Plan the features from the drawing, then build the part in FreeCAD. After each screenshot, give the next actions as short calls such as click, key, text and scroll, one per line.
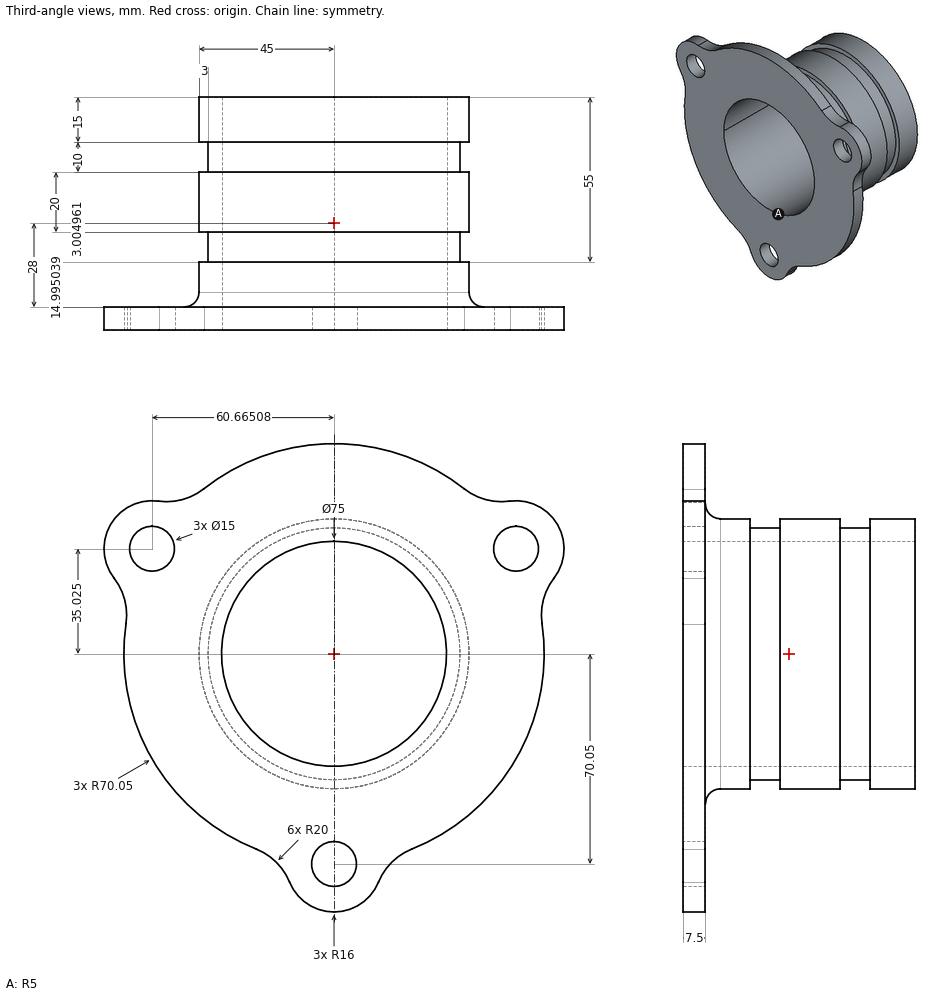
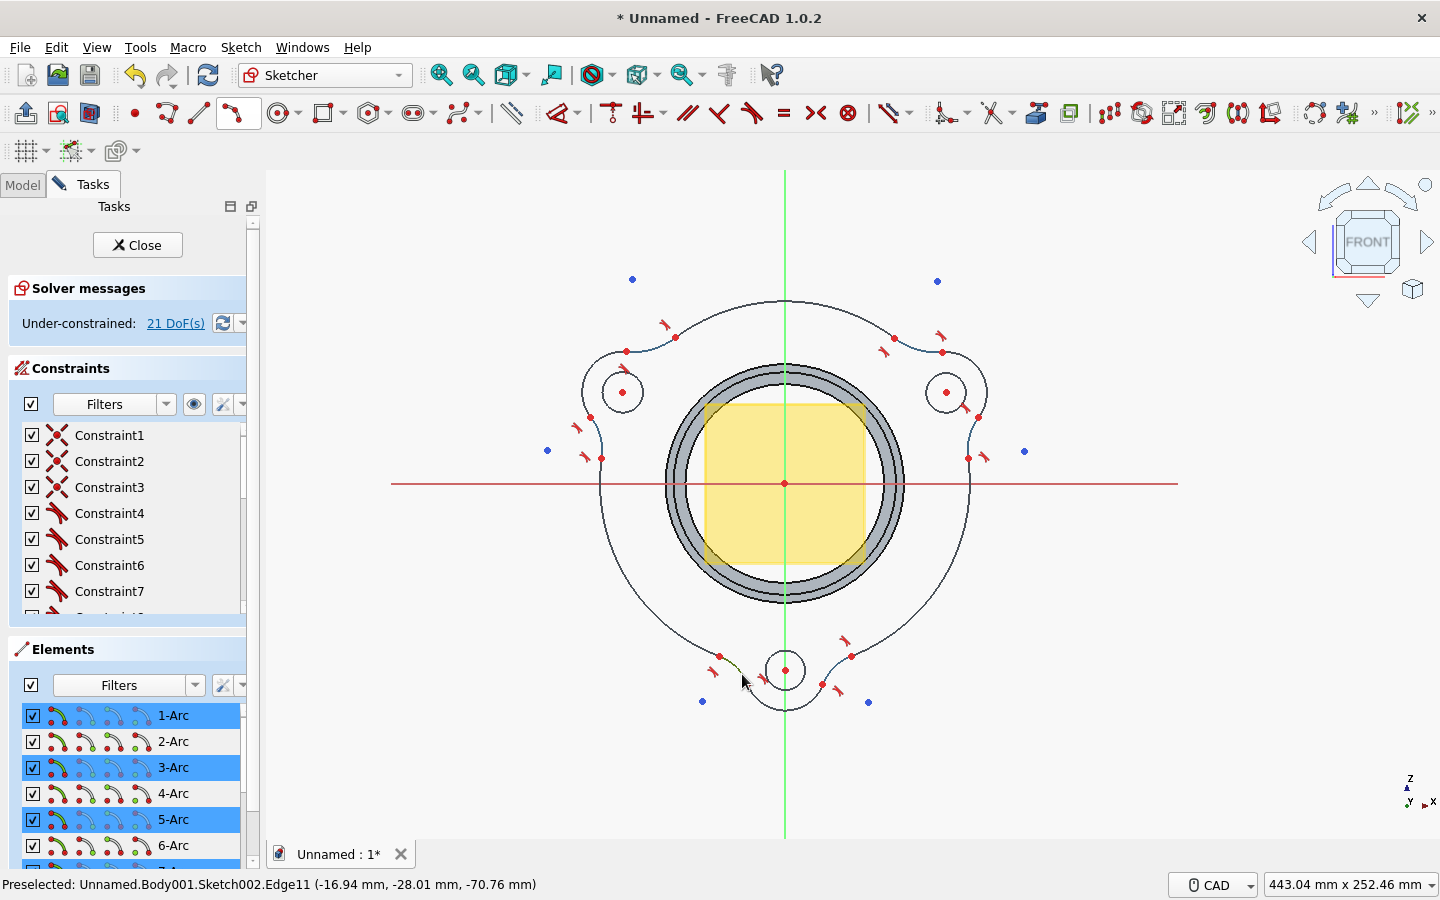
key(e)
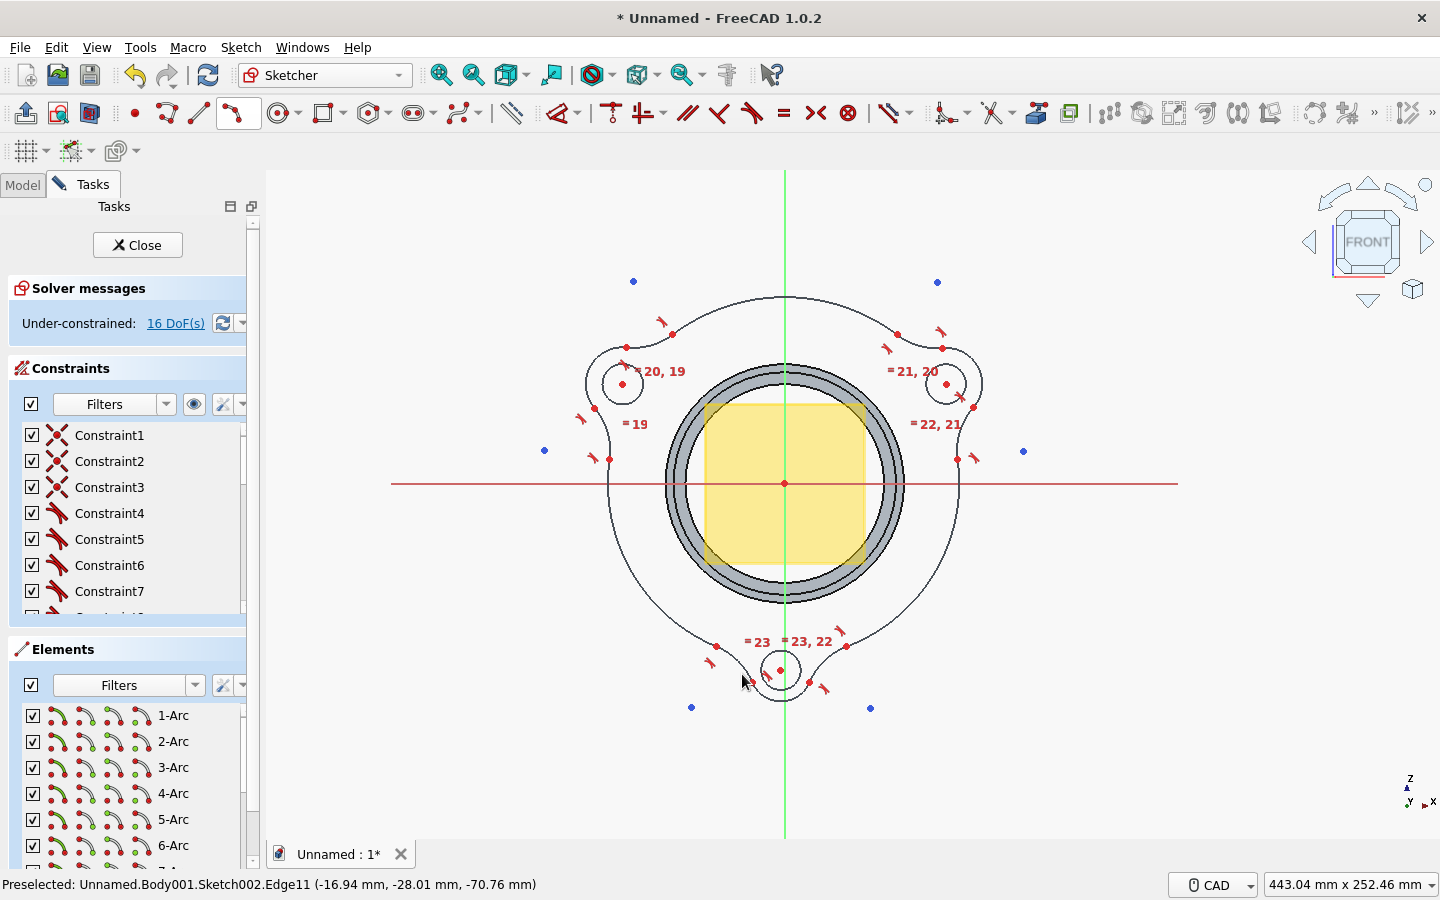
click(602, 354)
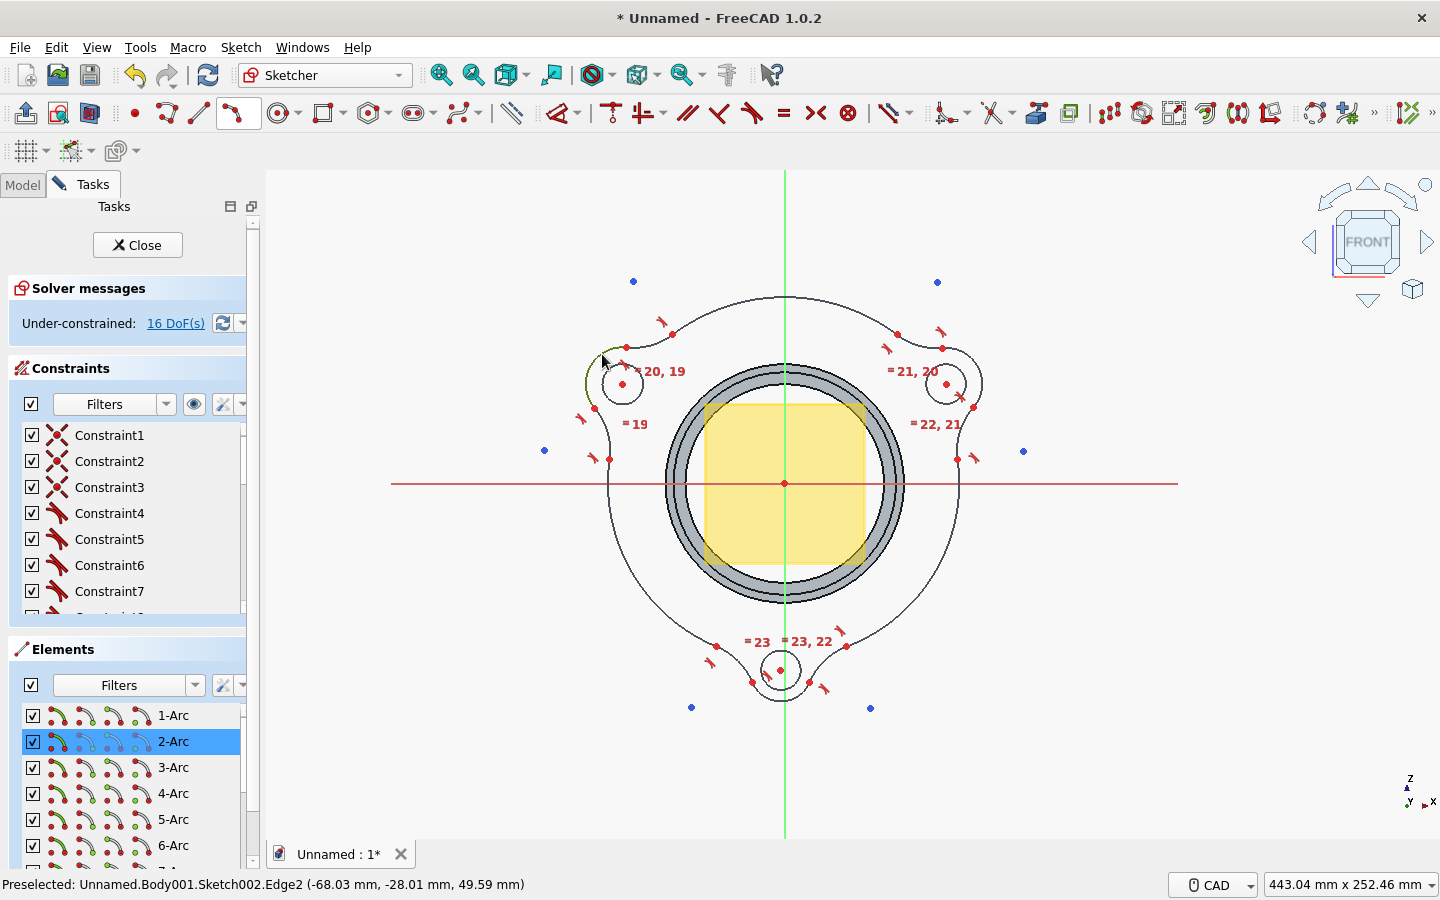
click(982, 384)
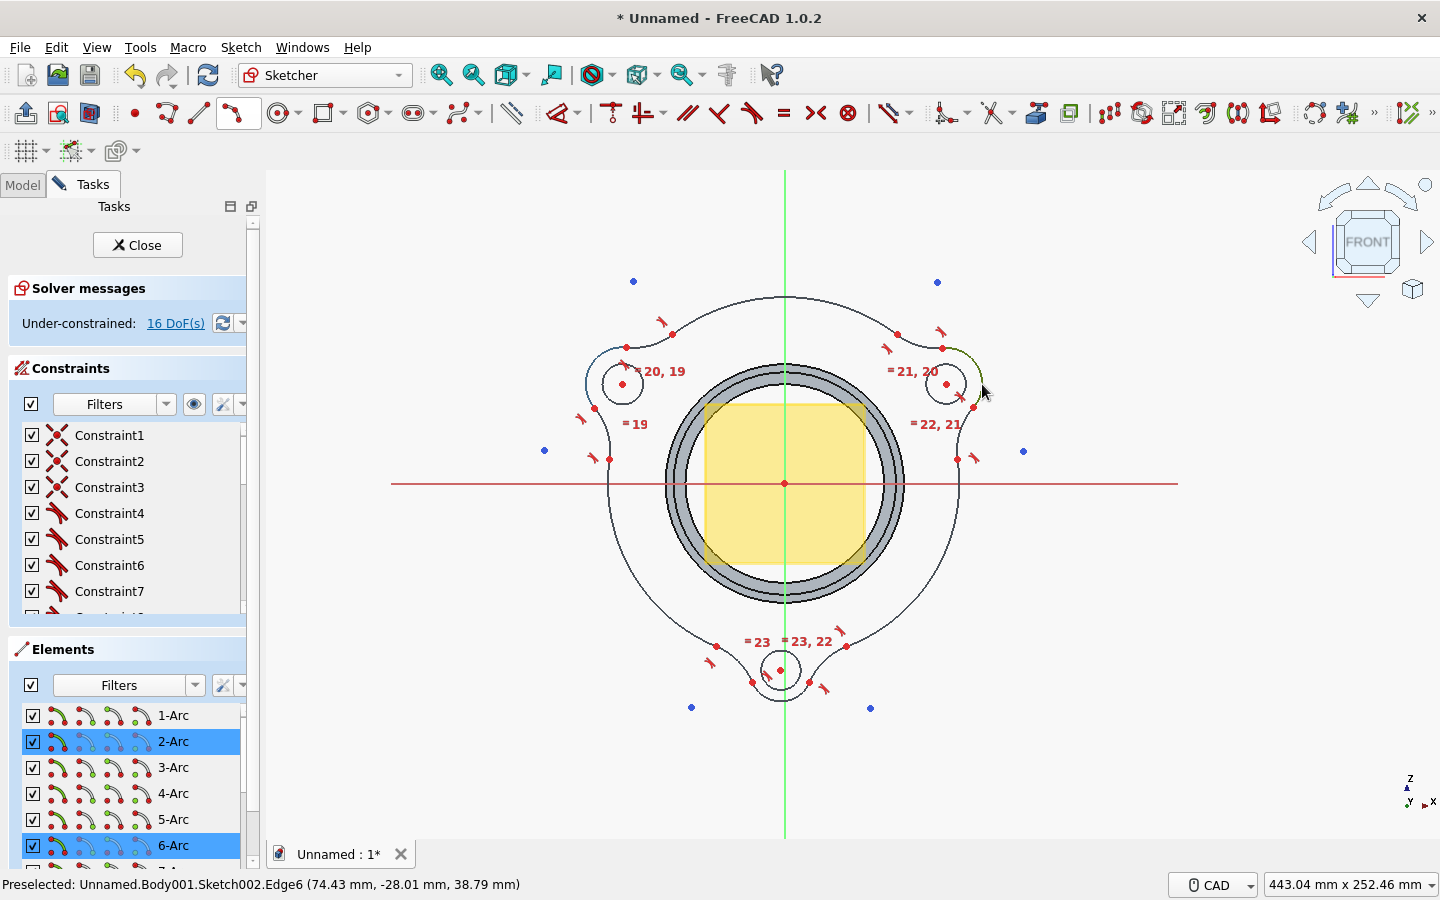
click(767, 698)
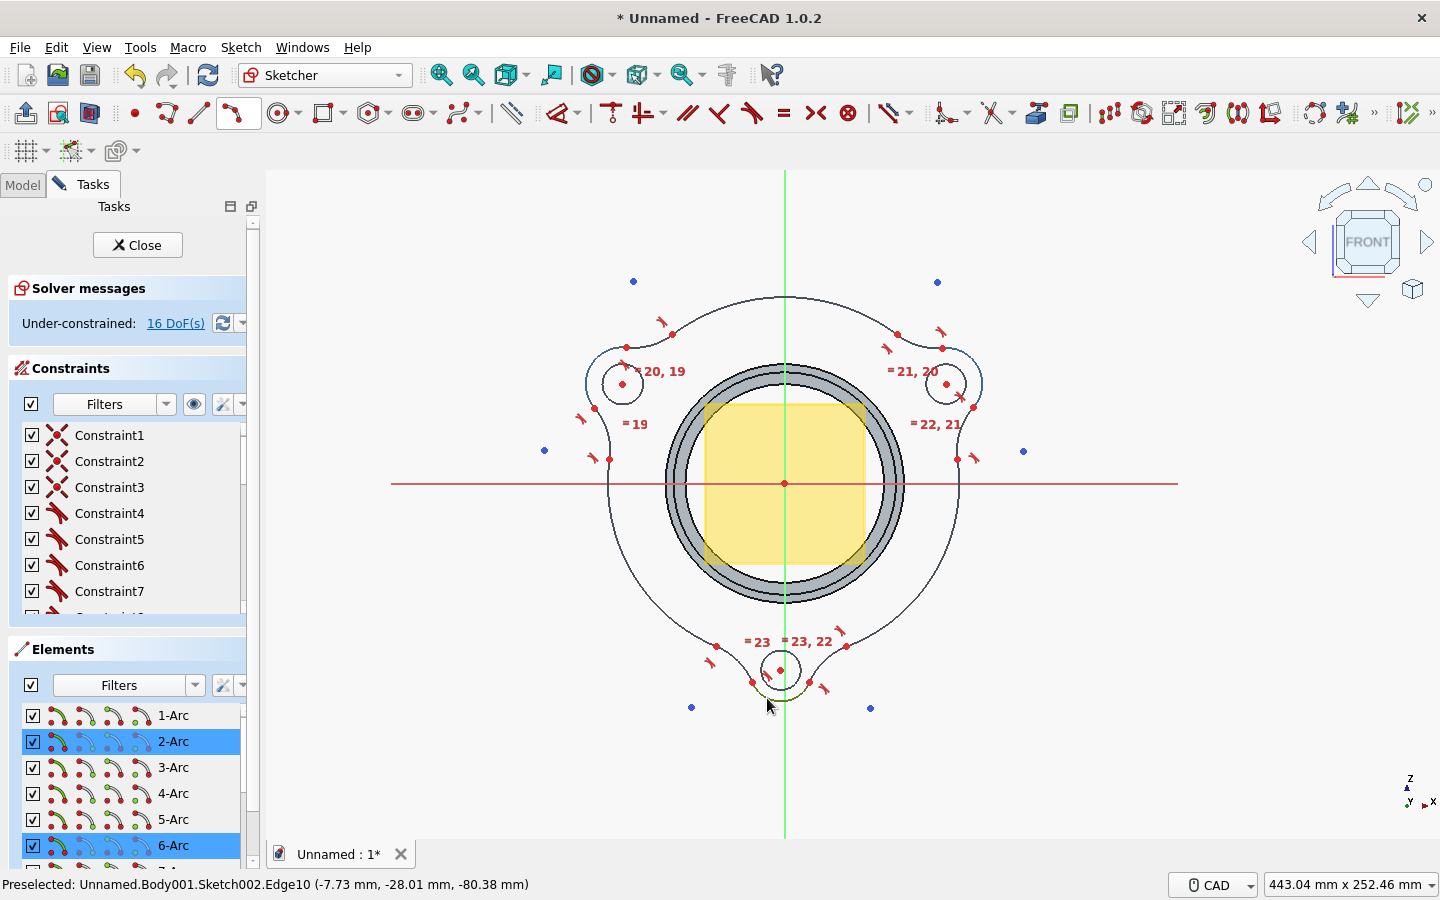
key(e)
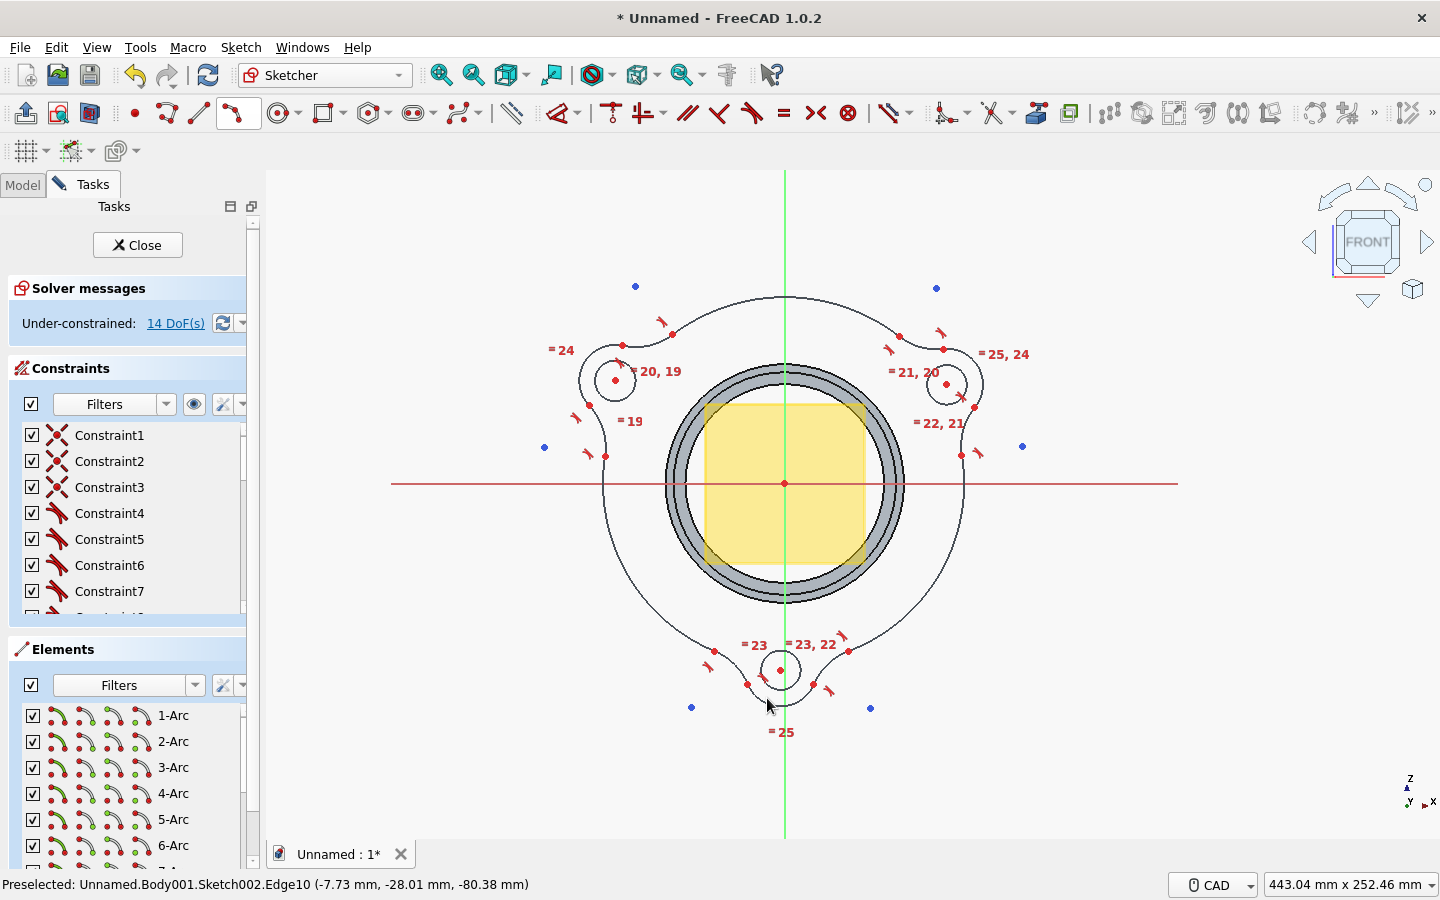
click(834, 304)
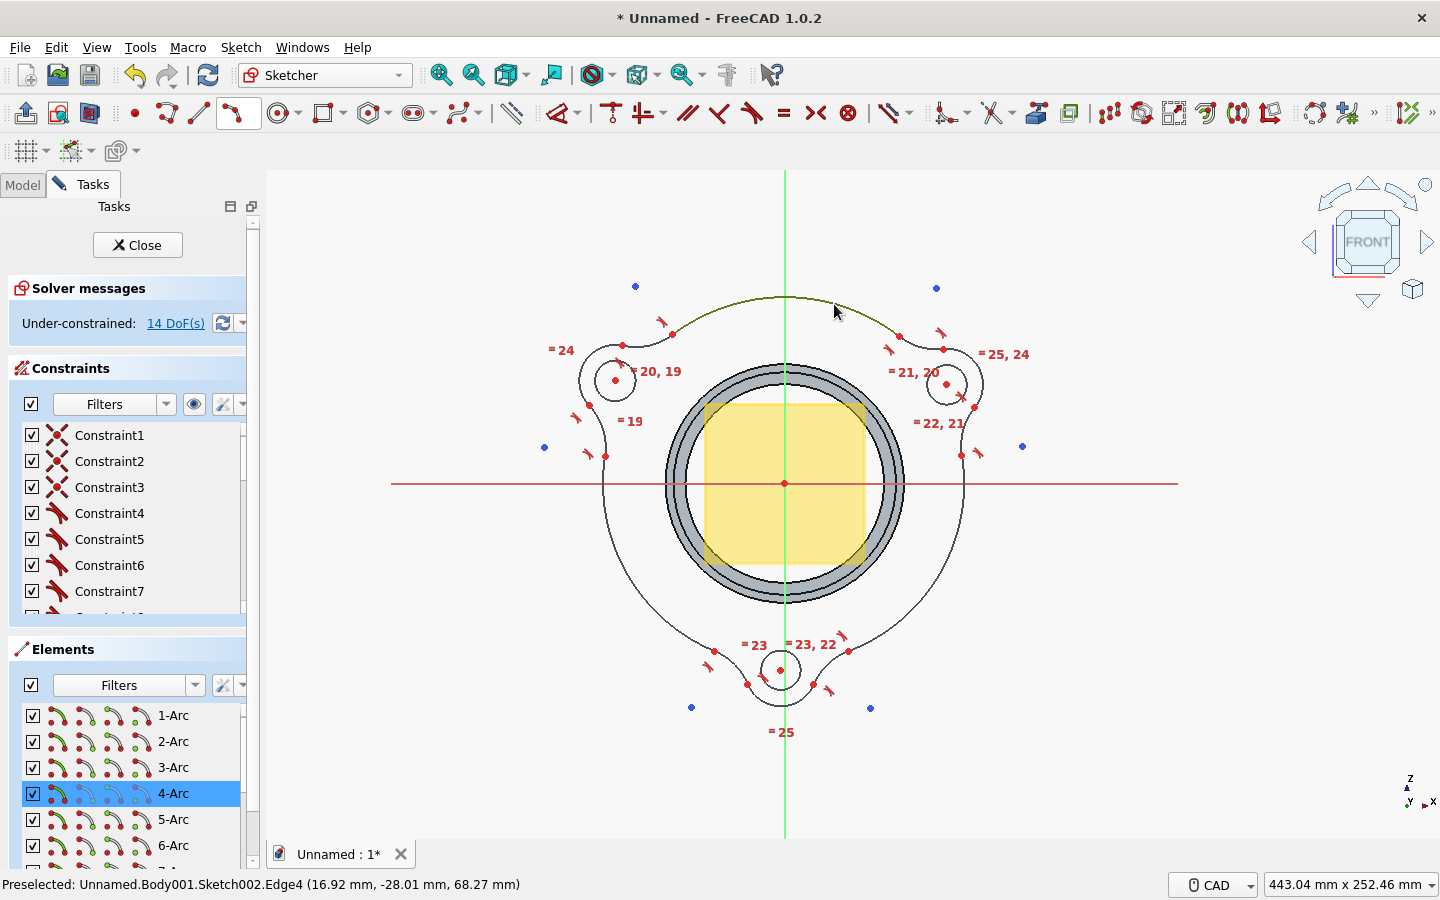
click(910, 612)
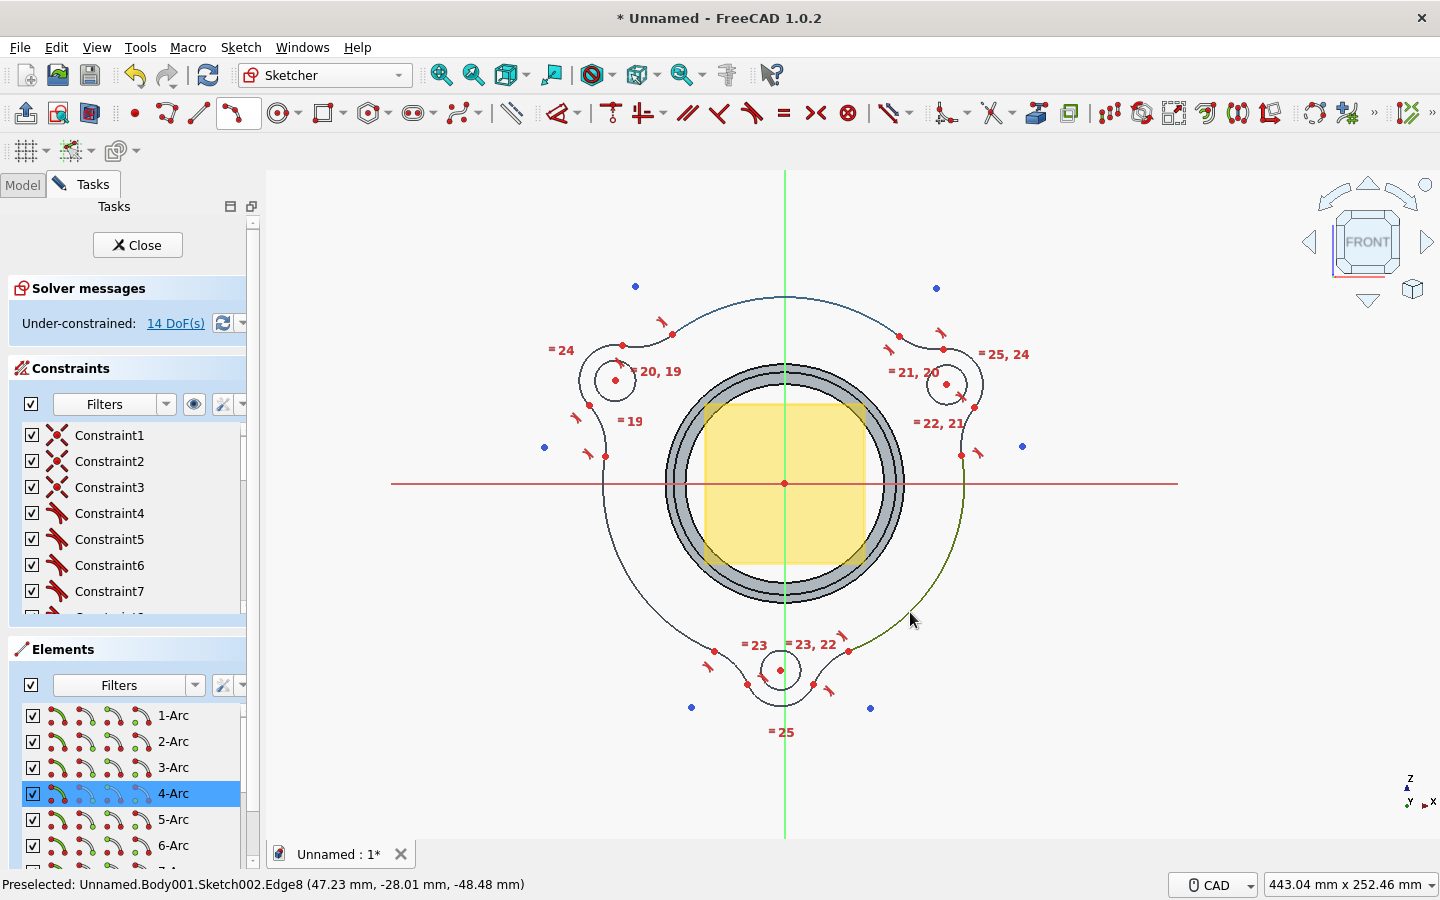
click(609, 528)